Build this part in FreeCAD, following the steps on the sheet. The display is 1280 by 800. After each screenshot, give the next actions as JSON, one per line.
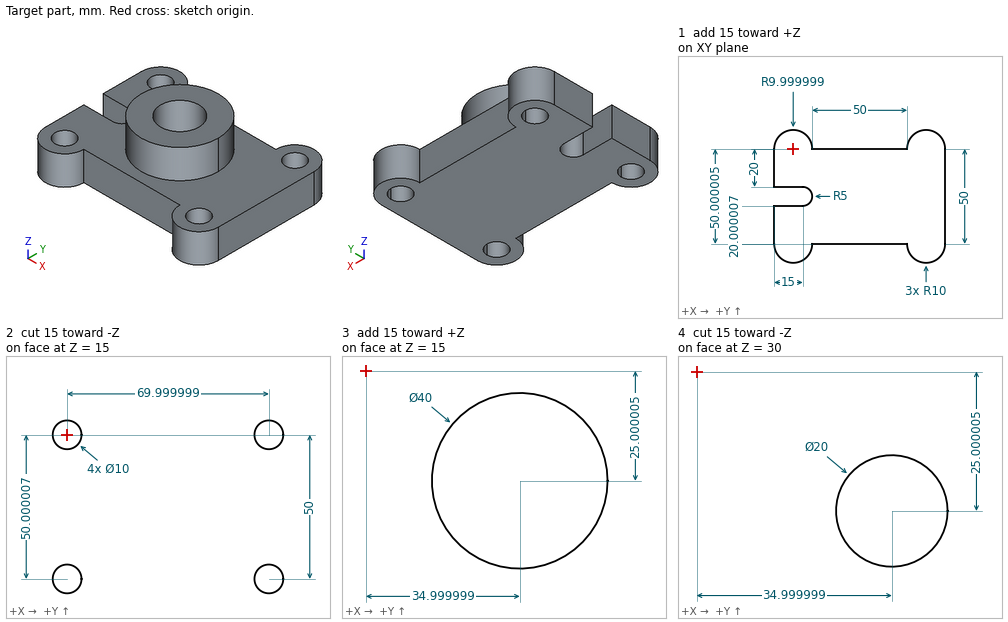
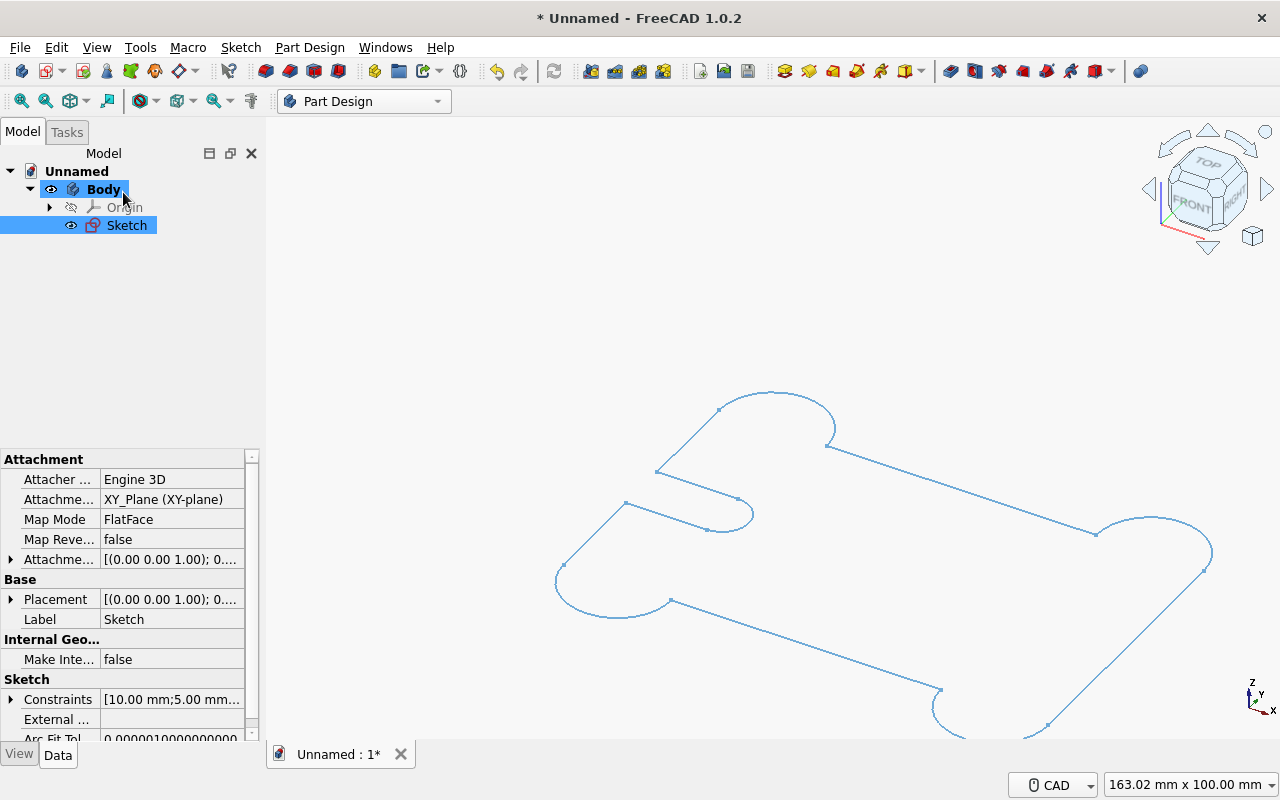
{"action": "left_click", "coordinate": [786, 72]}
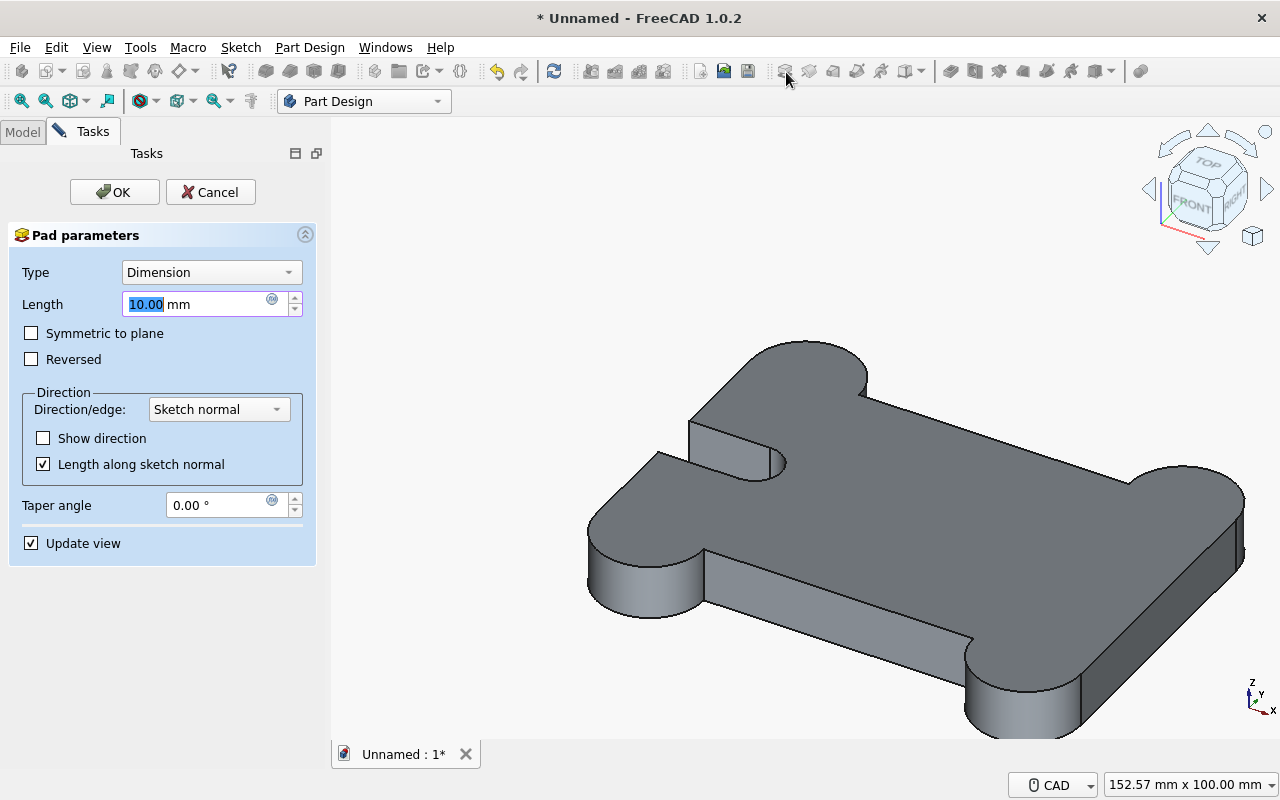
{"action": "type", "text": "15"}
{"action": "key", "text": "Tab"}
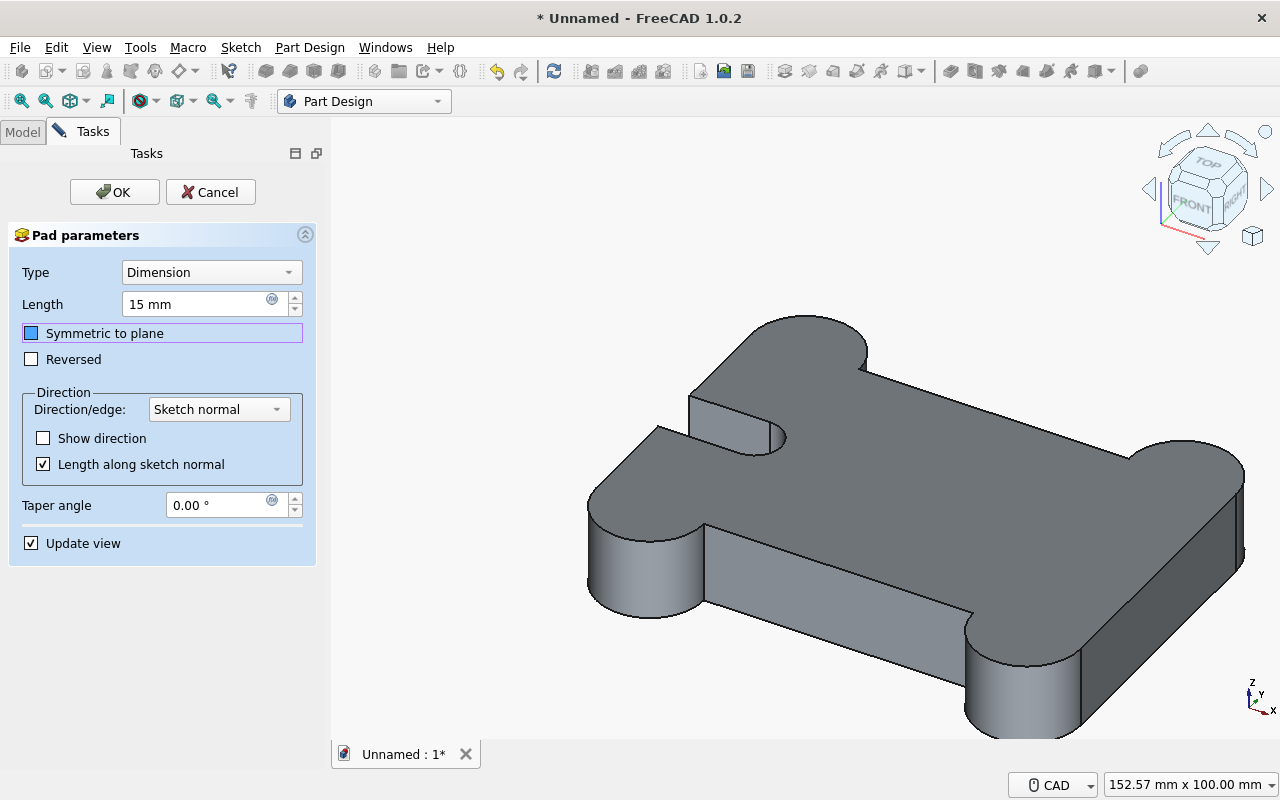
{"action": "left_click", "coordinate": [115, 192]}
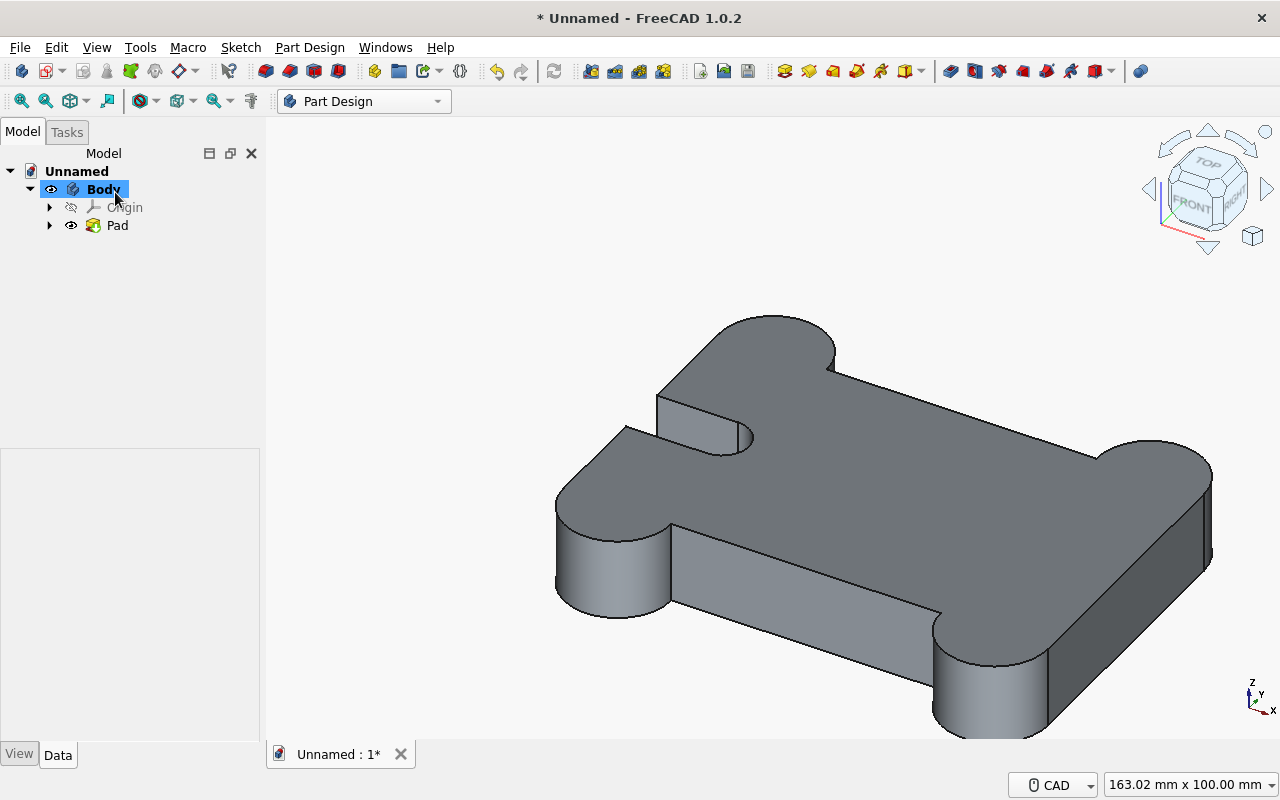
{"action": "left_click", "coordinate": [22, 102]}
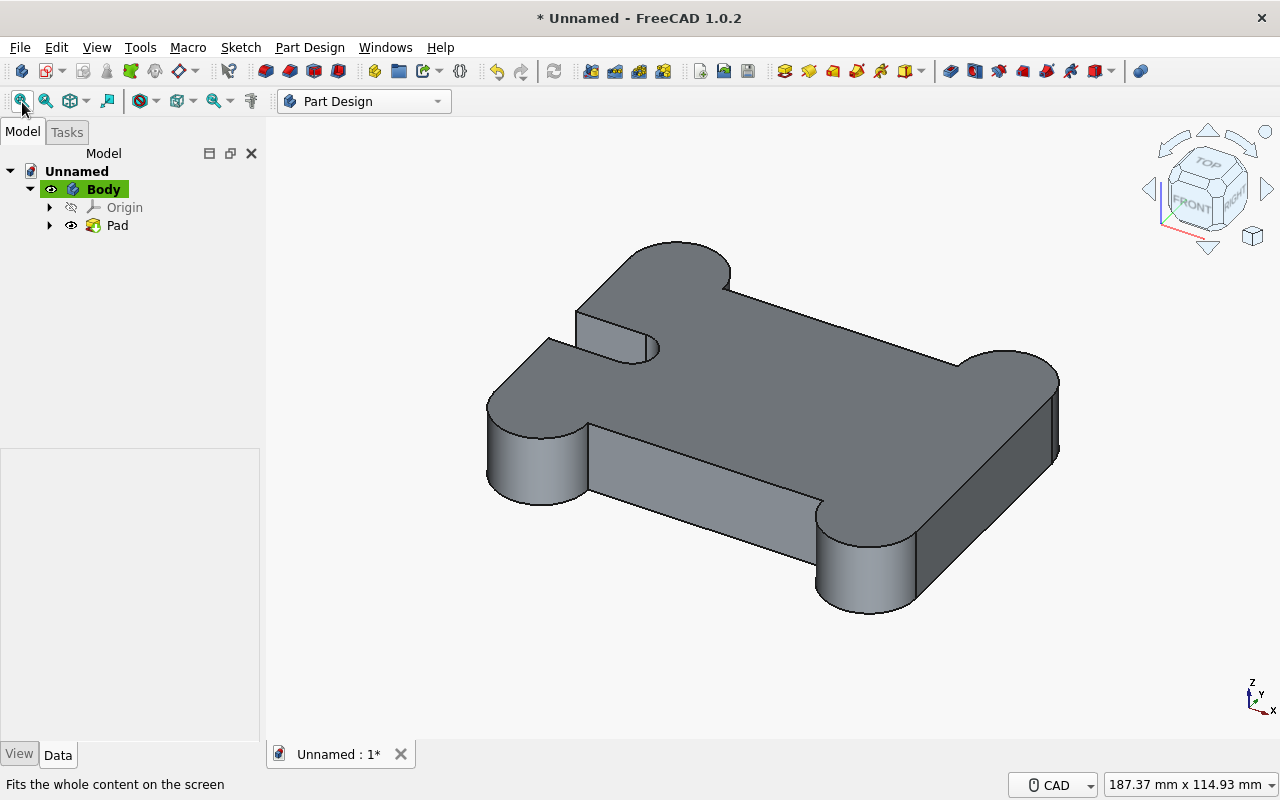
{"action": "left_click", "coordinate": [833, 414]}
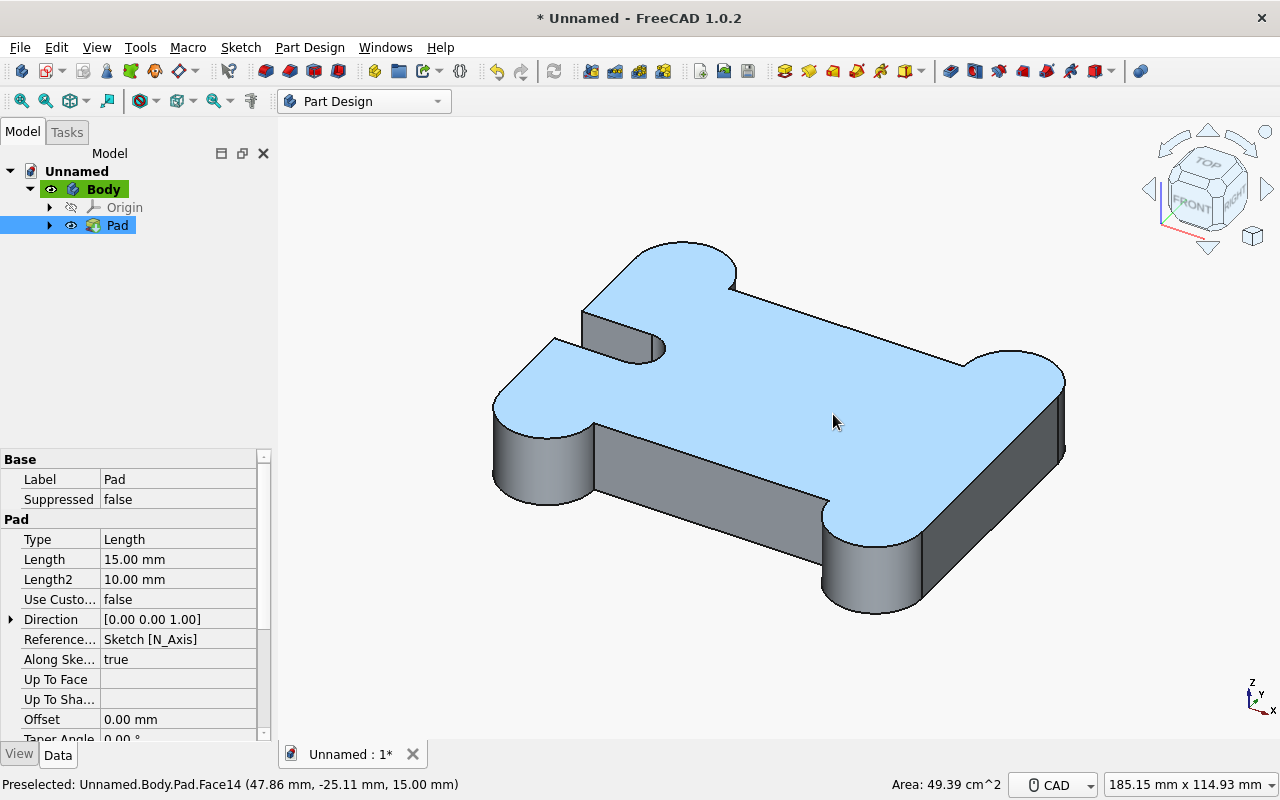
{"action": "left_click", "coordinate": [46, 72]}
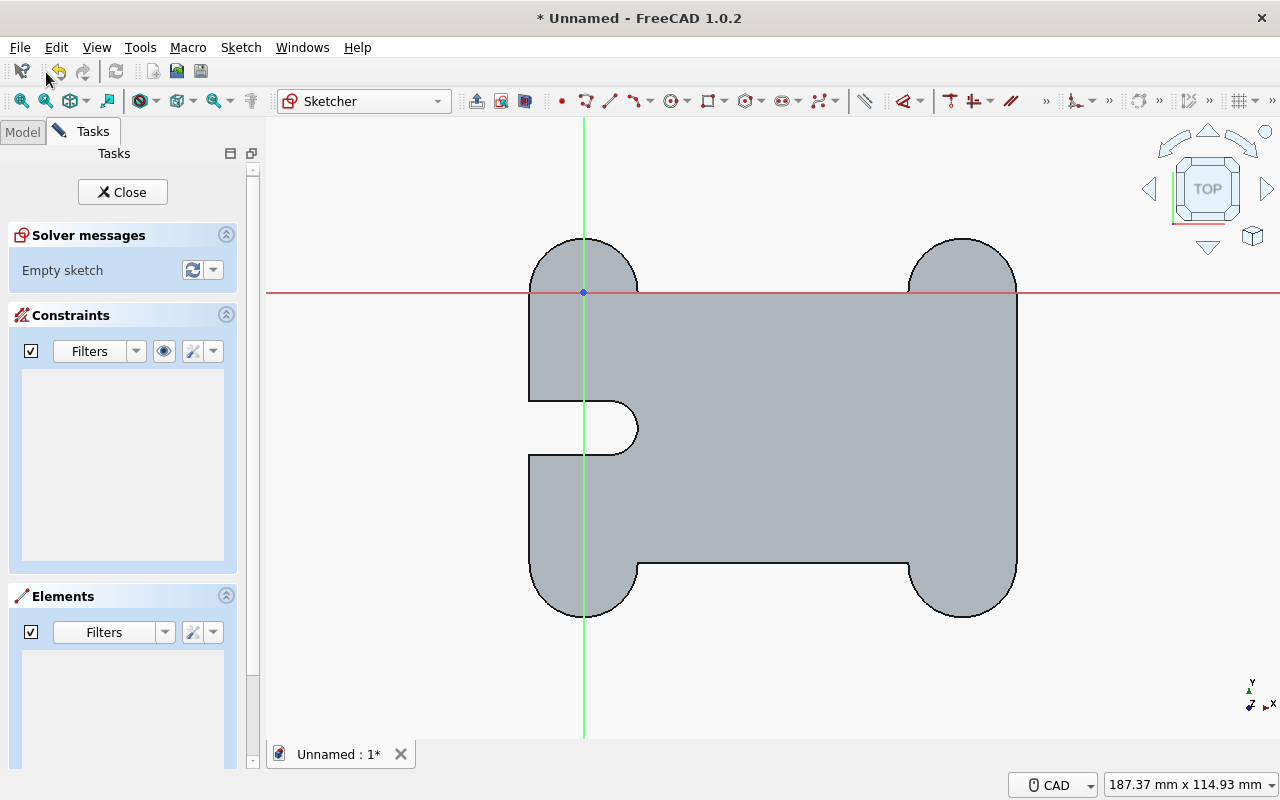
{"action": "left_click", "coordinate": [672, 102]}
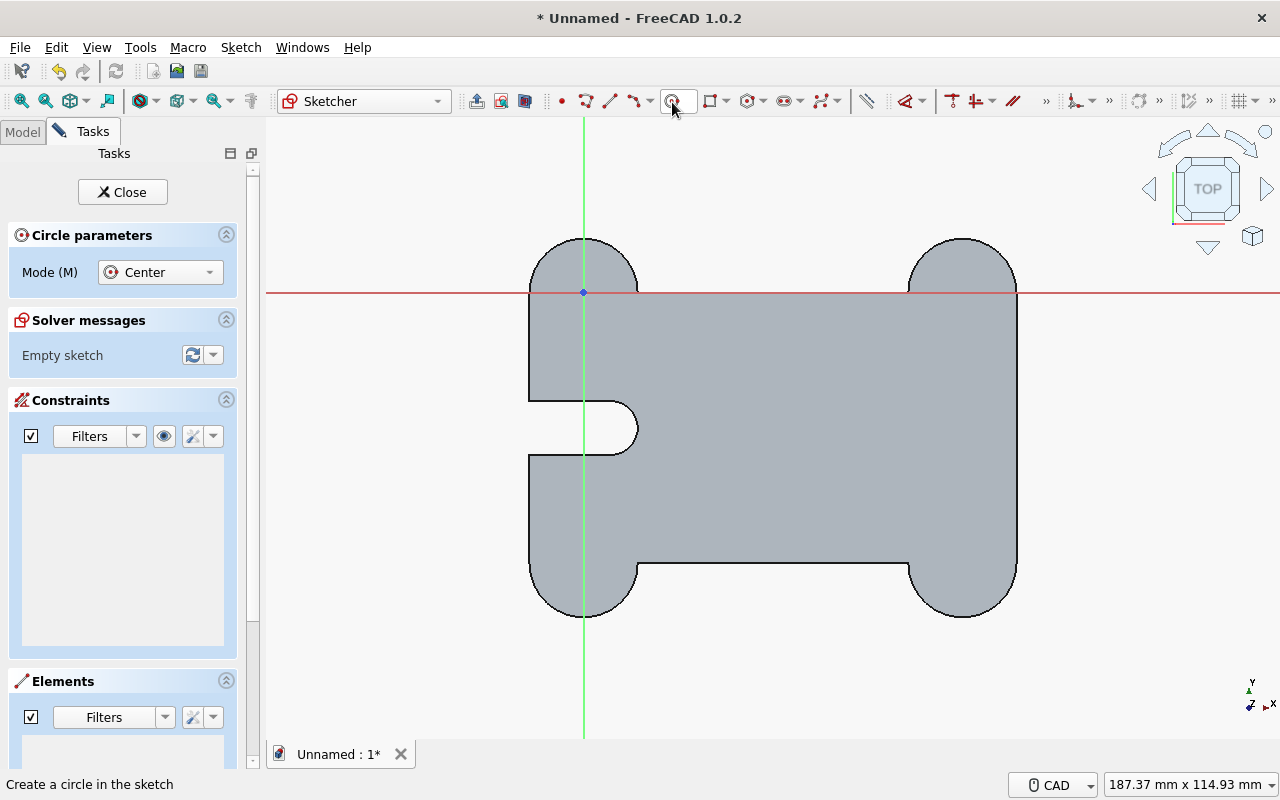
{"action": "left_click", "coordinate": [584, 293]}
{"action": "mouse_move", "coordinate": [603, 274]}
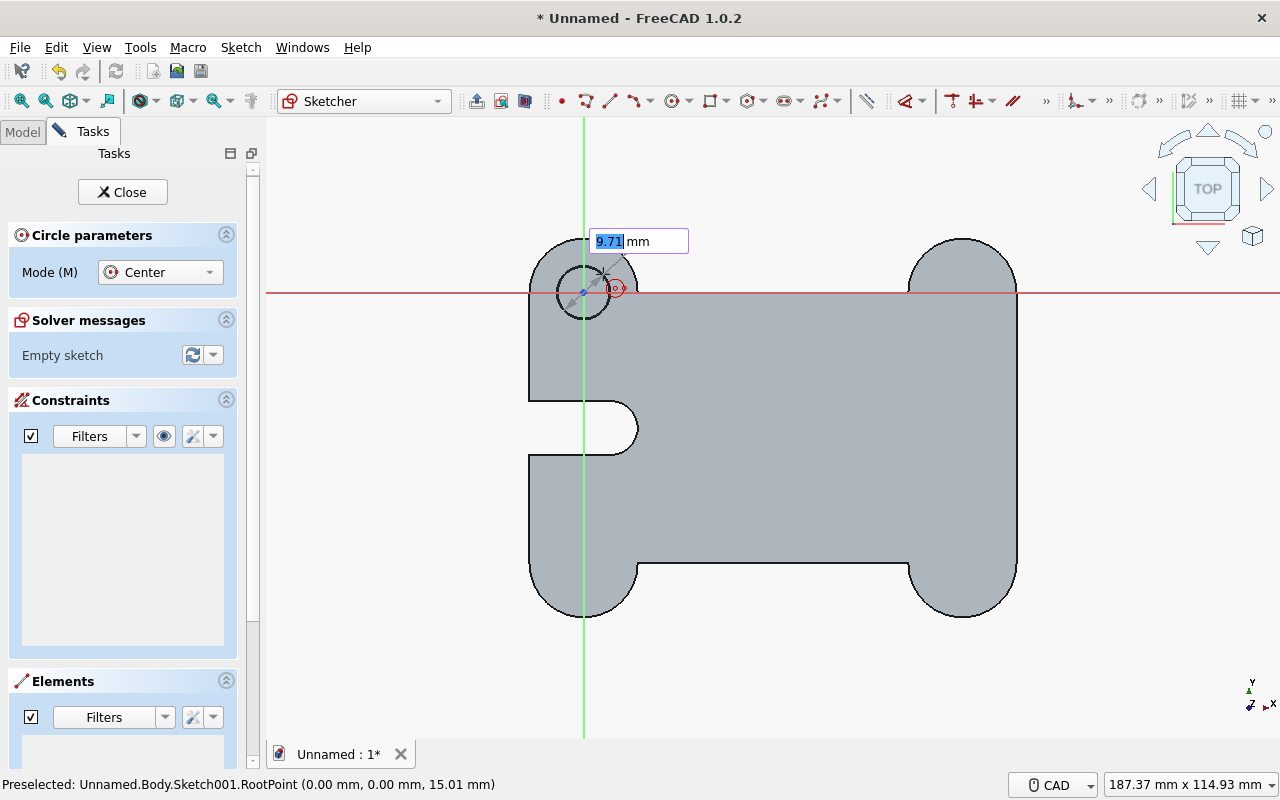
{"action": "type", "text": "10"}
{"action": "key", "text": "Return"}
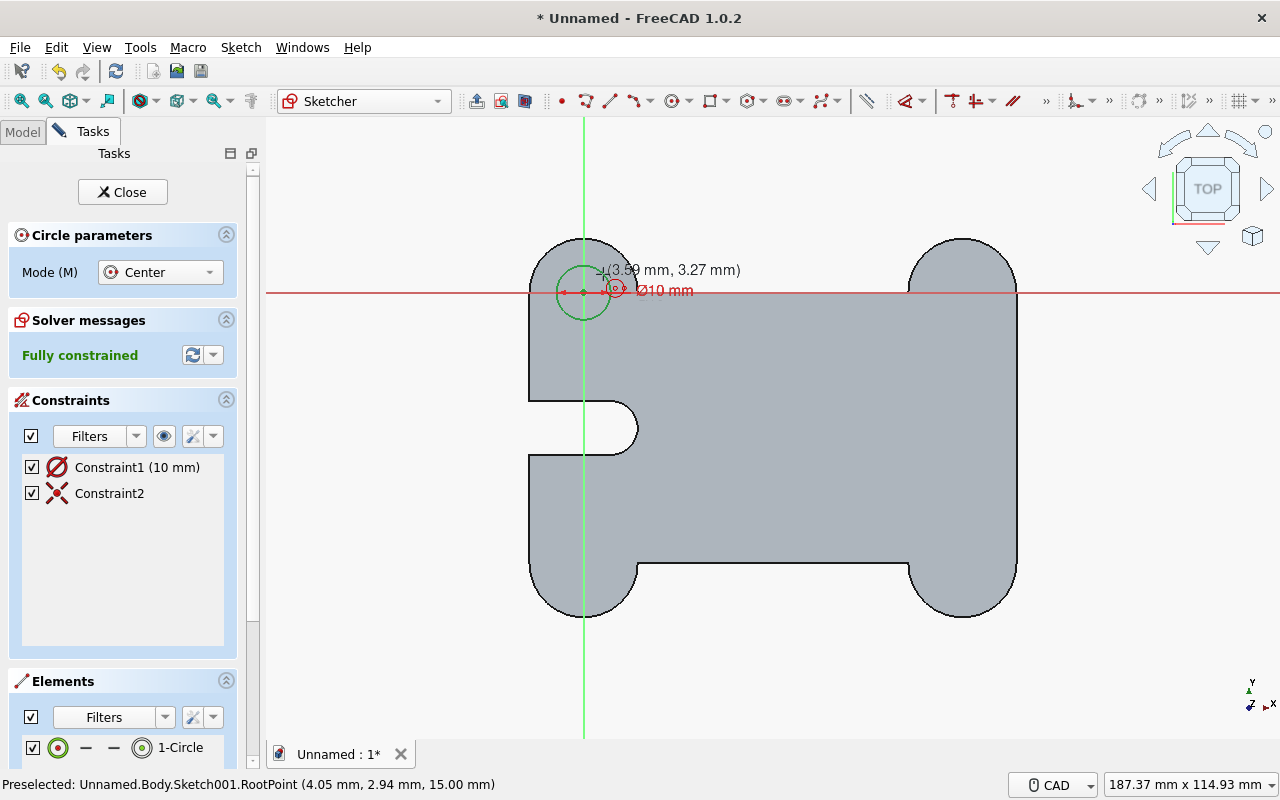
{"action": "left_click", "coordinate": [962, 293]}
{"action": "mouse_move", "coordinate": [982, 274]}